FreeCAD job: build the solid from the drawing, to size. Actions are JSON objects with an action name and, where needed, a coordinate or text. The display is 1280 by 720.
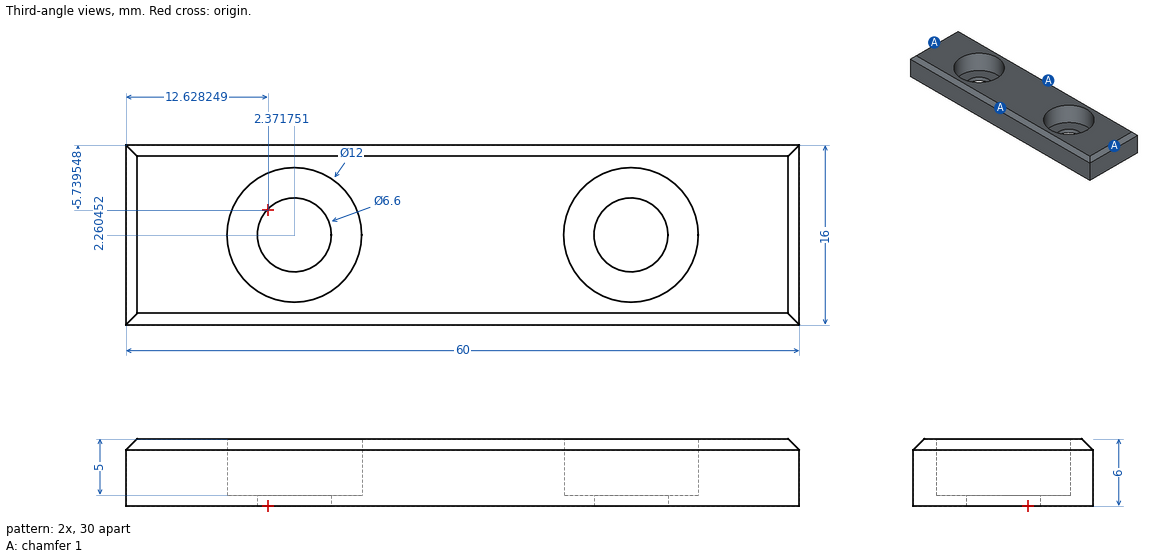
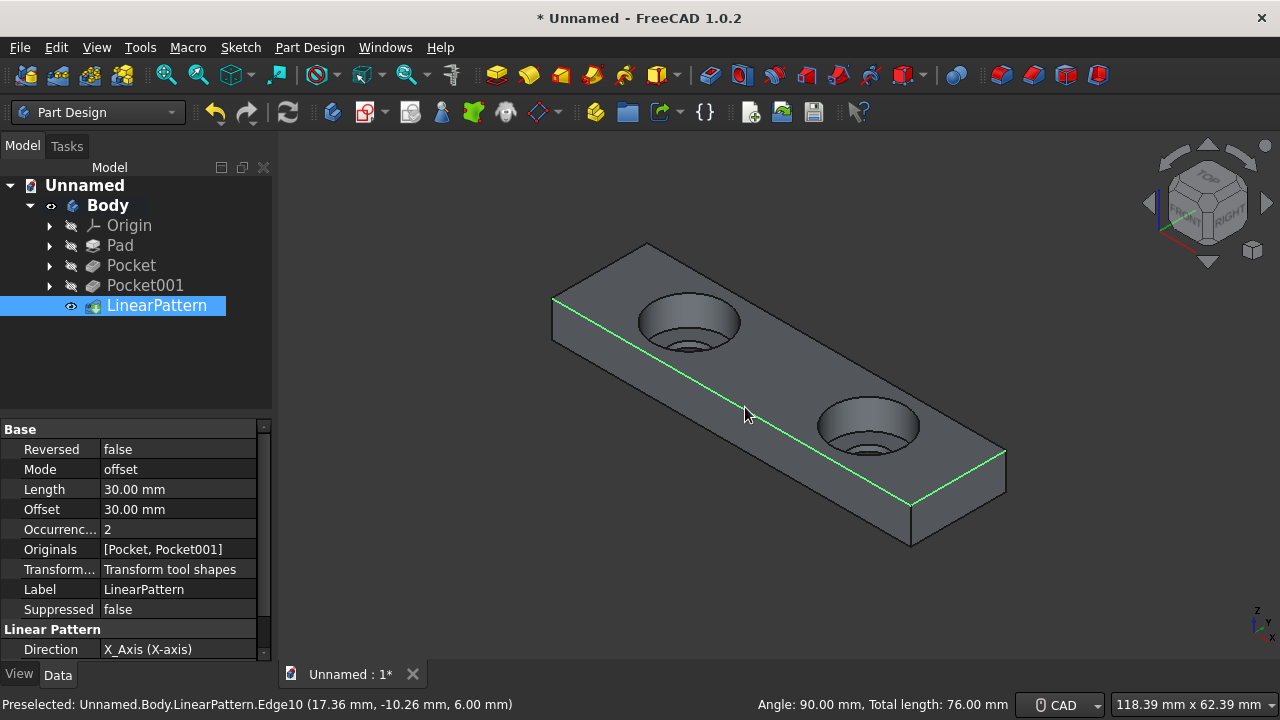
{"action": "key", "text": "2"}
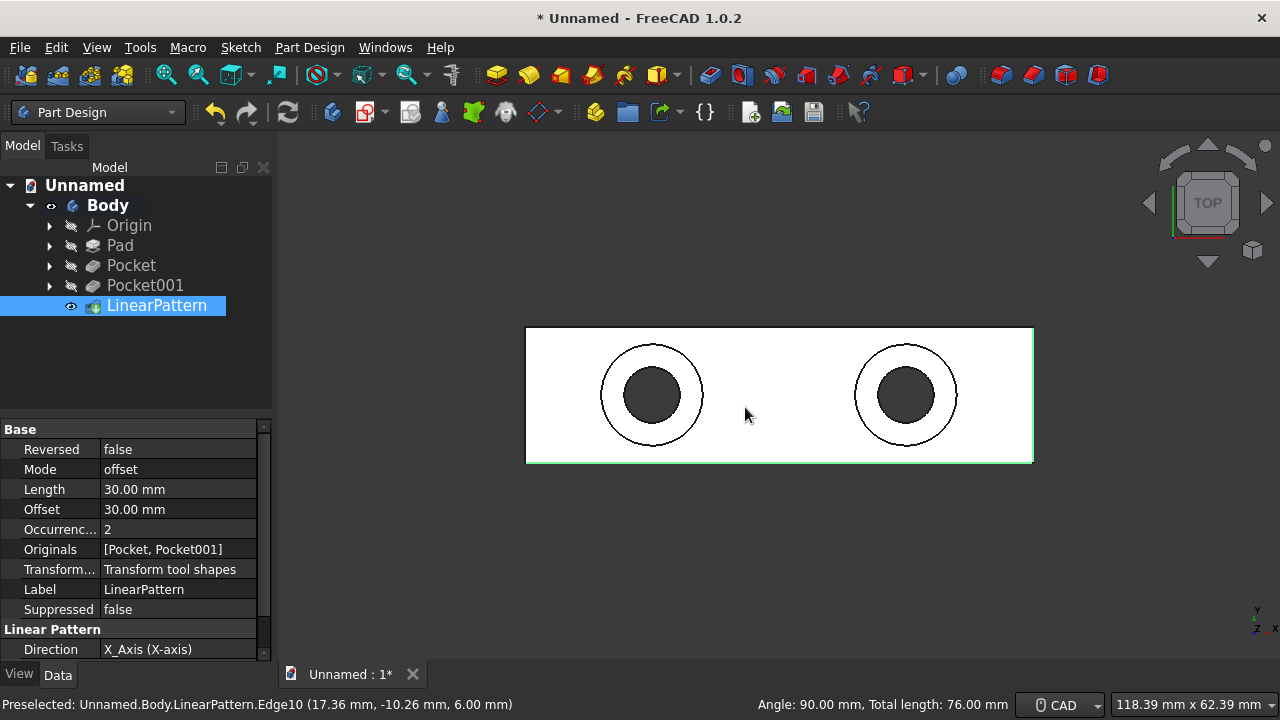
{"action": "left_click", "coordinate": [779, 326], "text": "ctrl"}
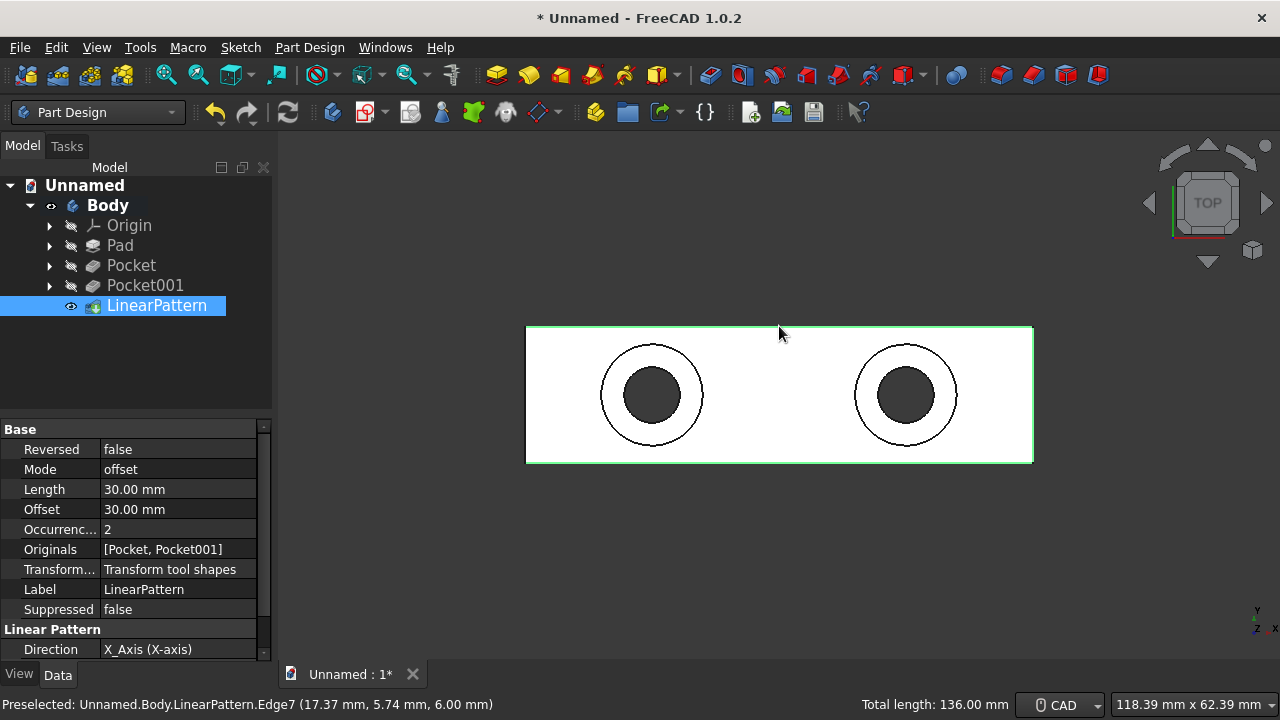
{"action": "left_click", "coordinate": [525, 394], "text": "ctrl"}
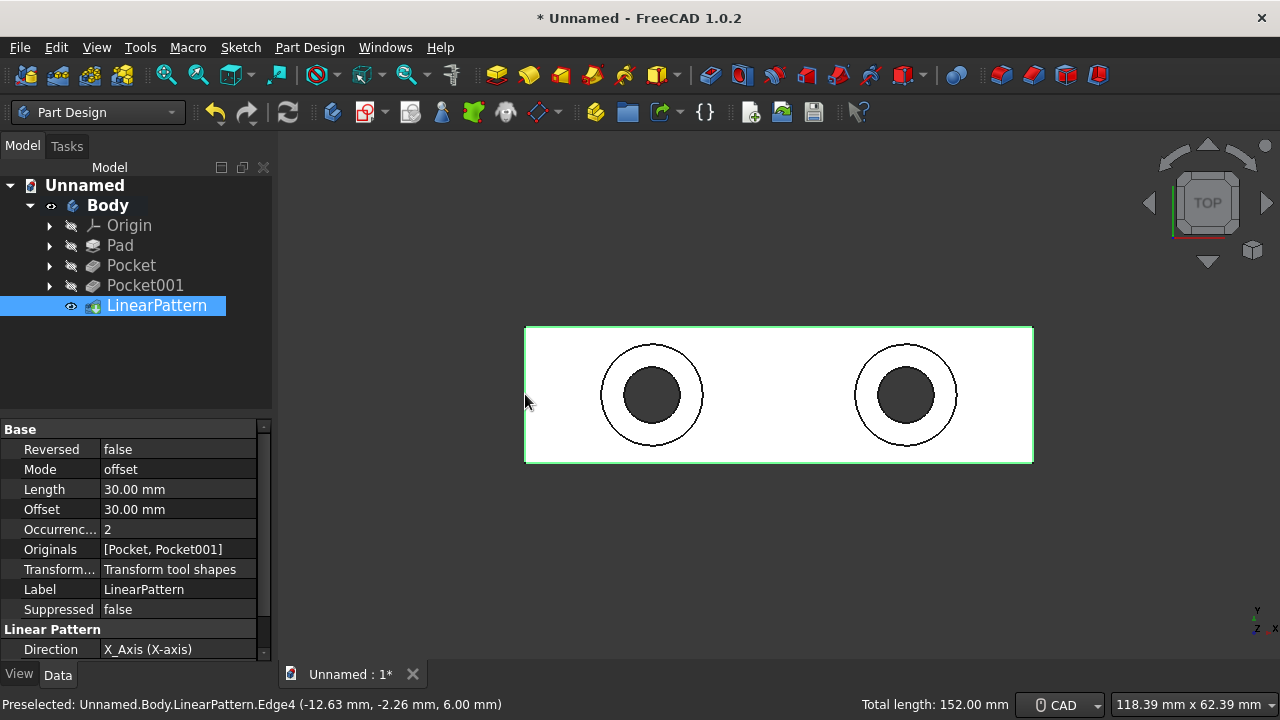
{"action": "left_click", "coordinate": [1034, 76]}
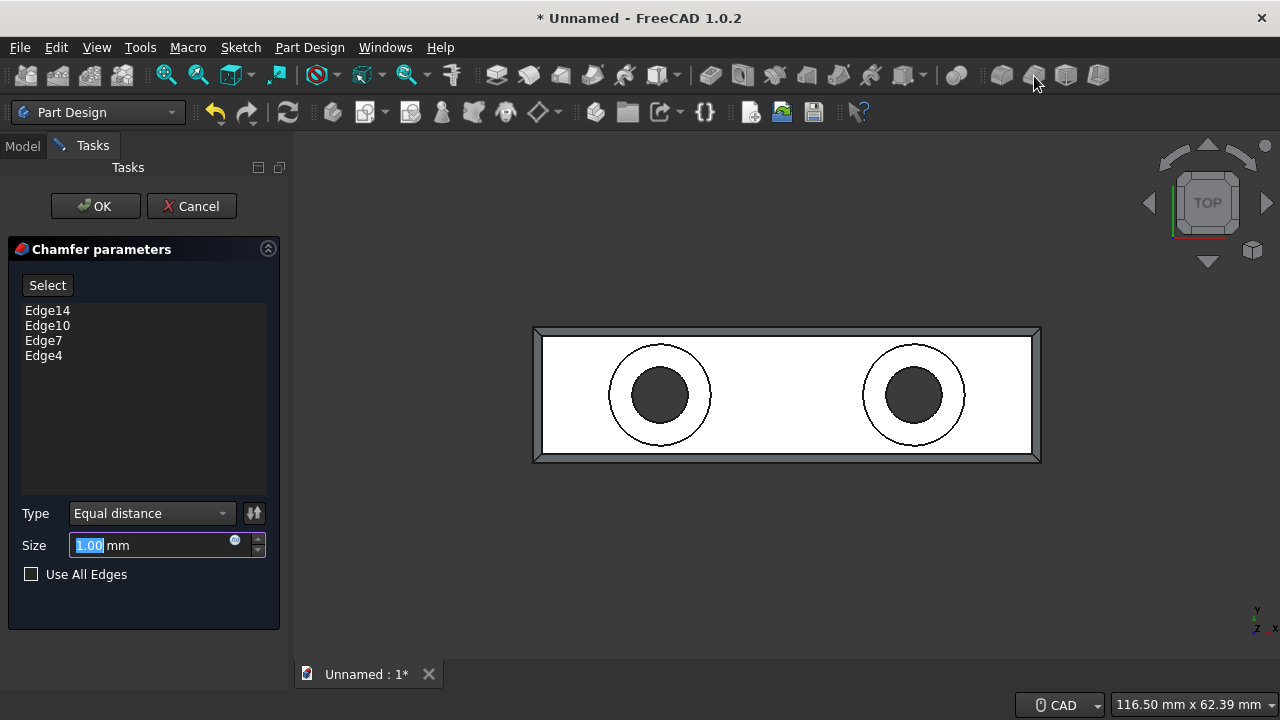
{"action": "type", "text": "1"}
{"action": "key", "text": "Tab"}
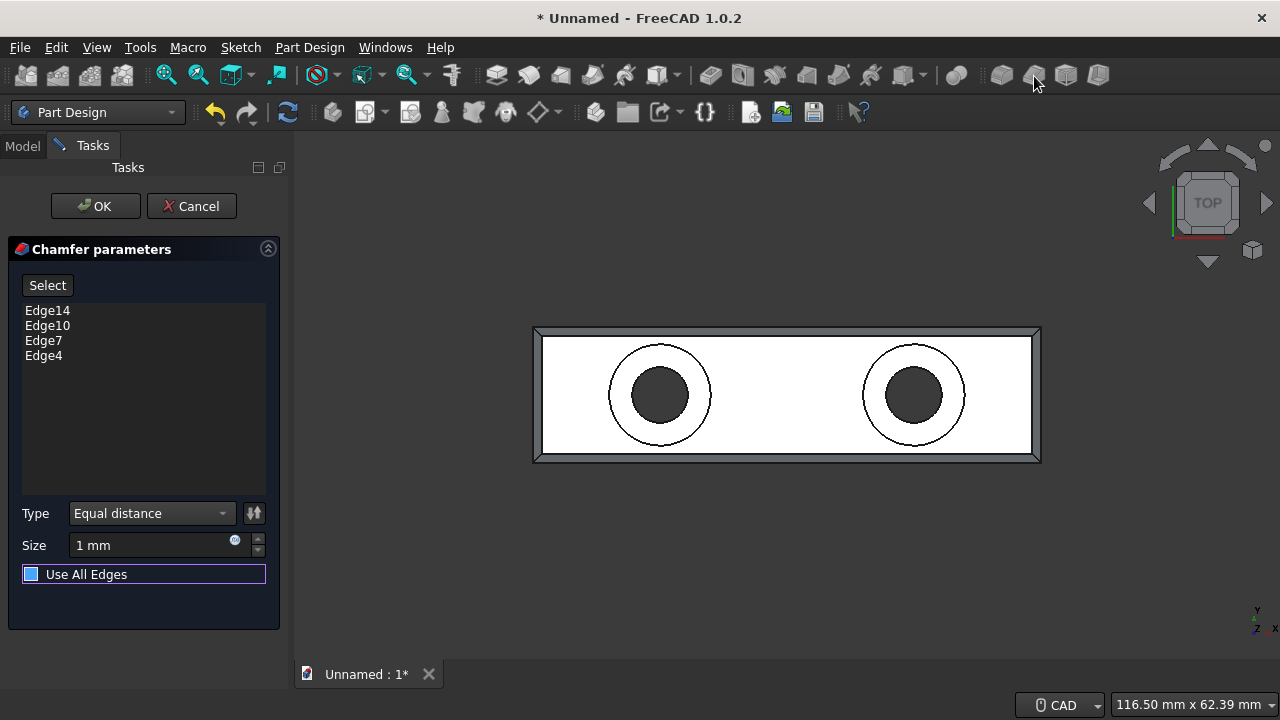
{"action": "left_click", "coordinate": [96, 206]}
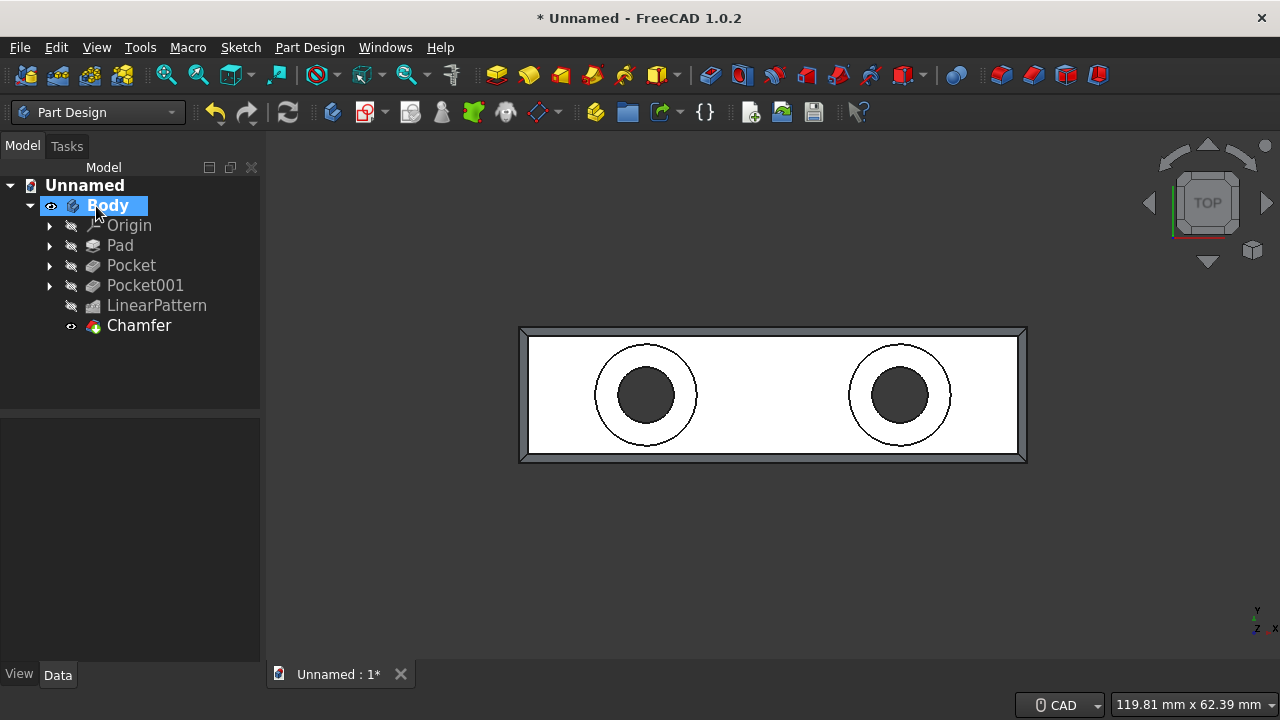
{"action": "key", "text": "0"}